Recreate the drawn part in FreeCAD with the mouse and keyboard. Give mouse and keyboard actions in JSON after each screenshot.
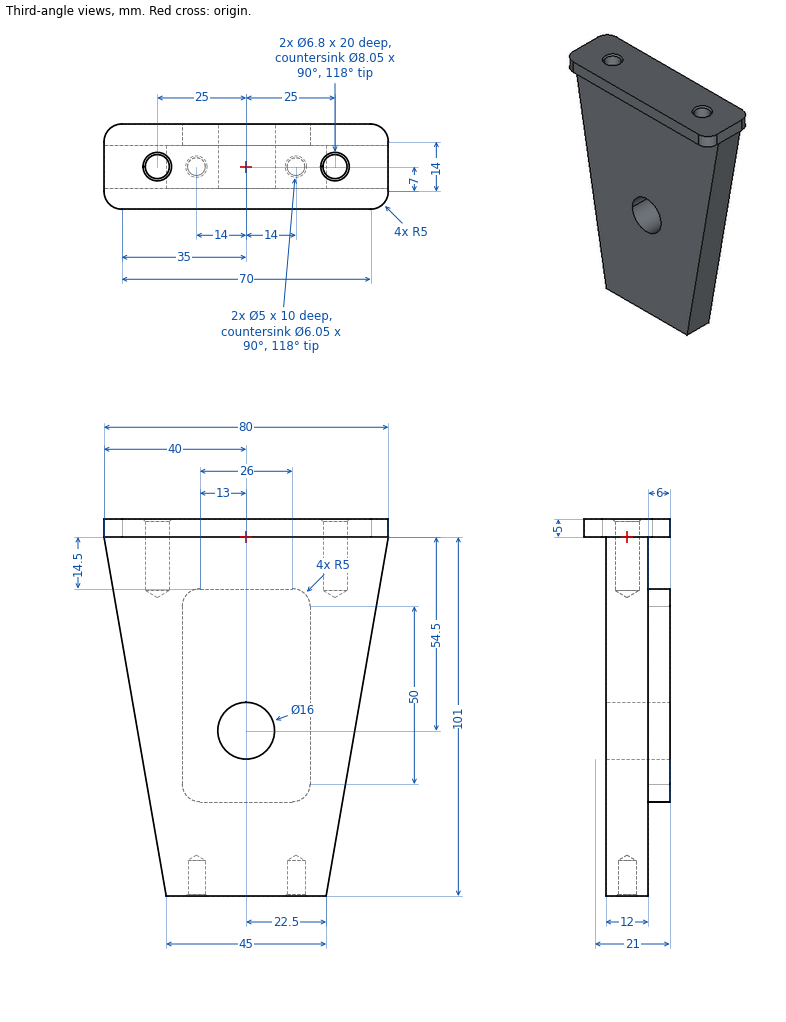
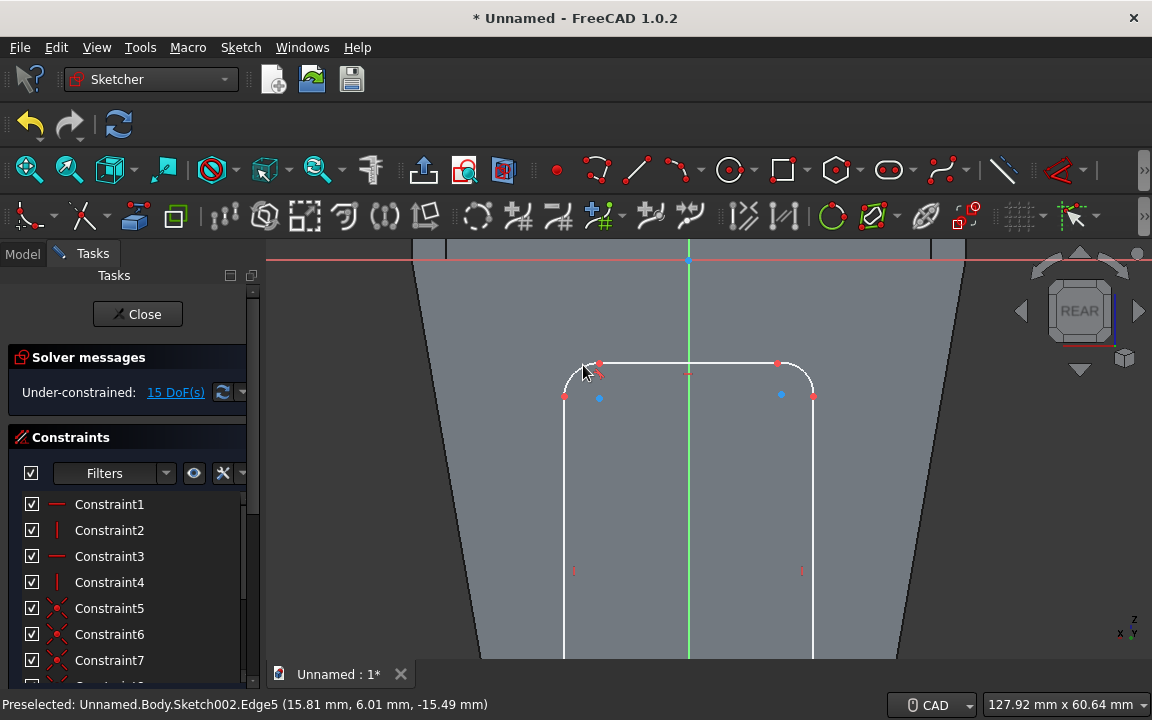
{"action": "left_click", "coordinate": [724, 363]}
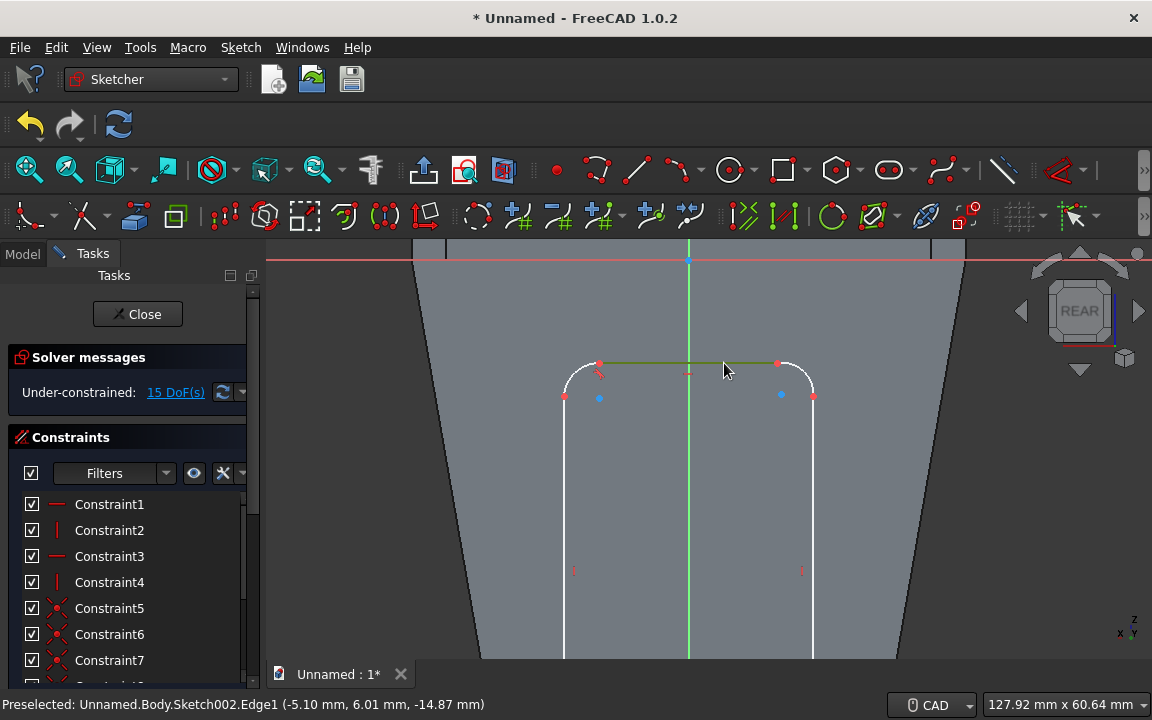
{"action": "left_click", "coordinate": [810, 380]}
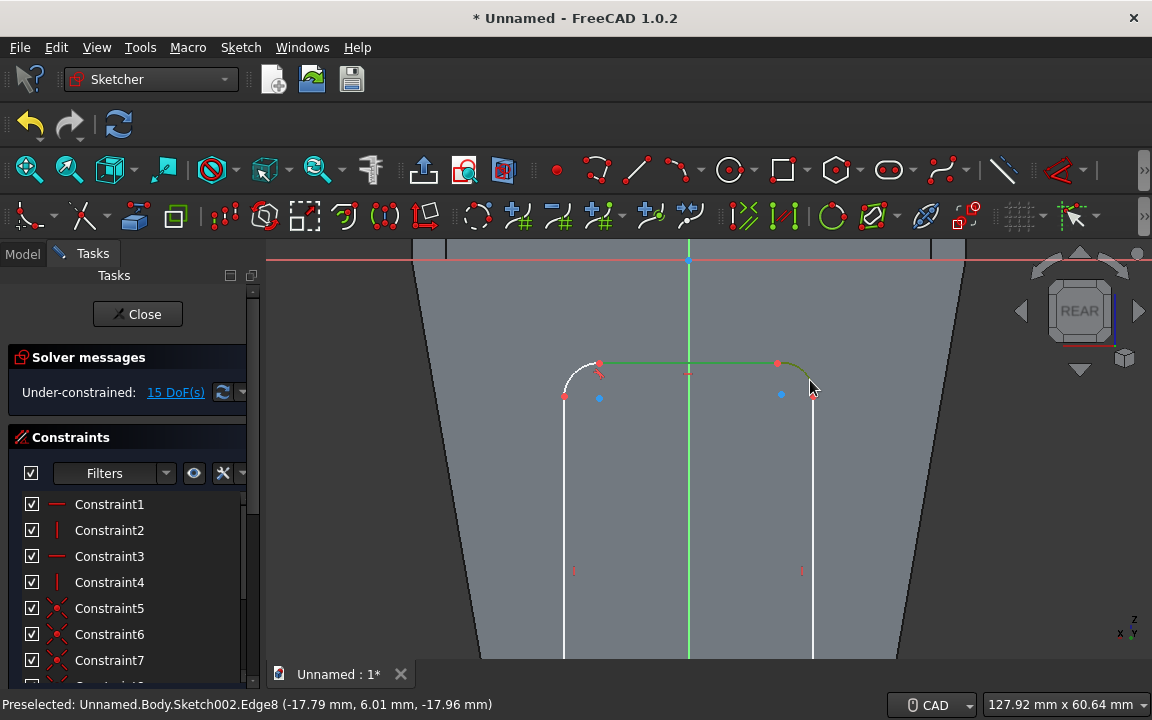
{"action": "key", "text": "t"}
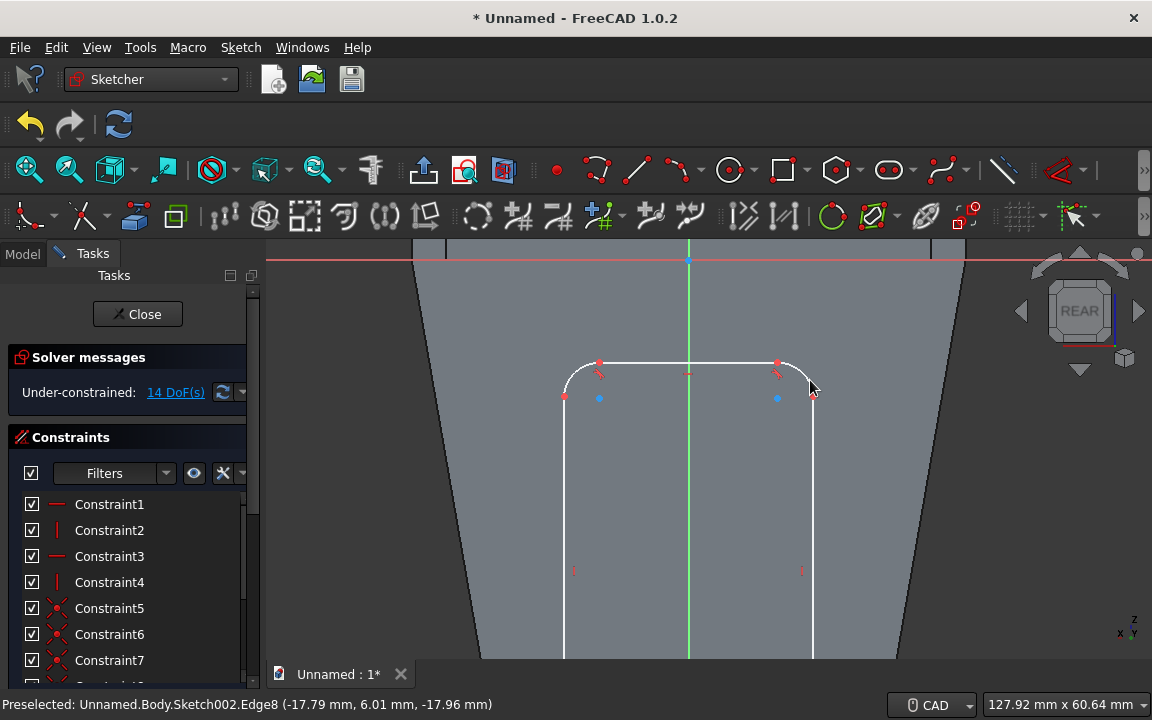
{"action": "left_click", "coordinate": [564, 501]}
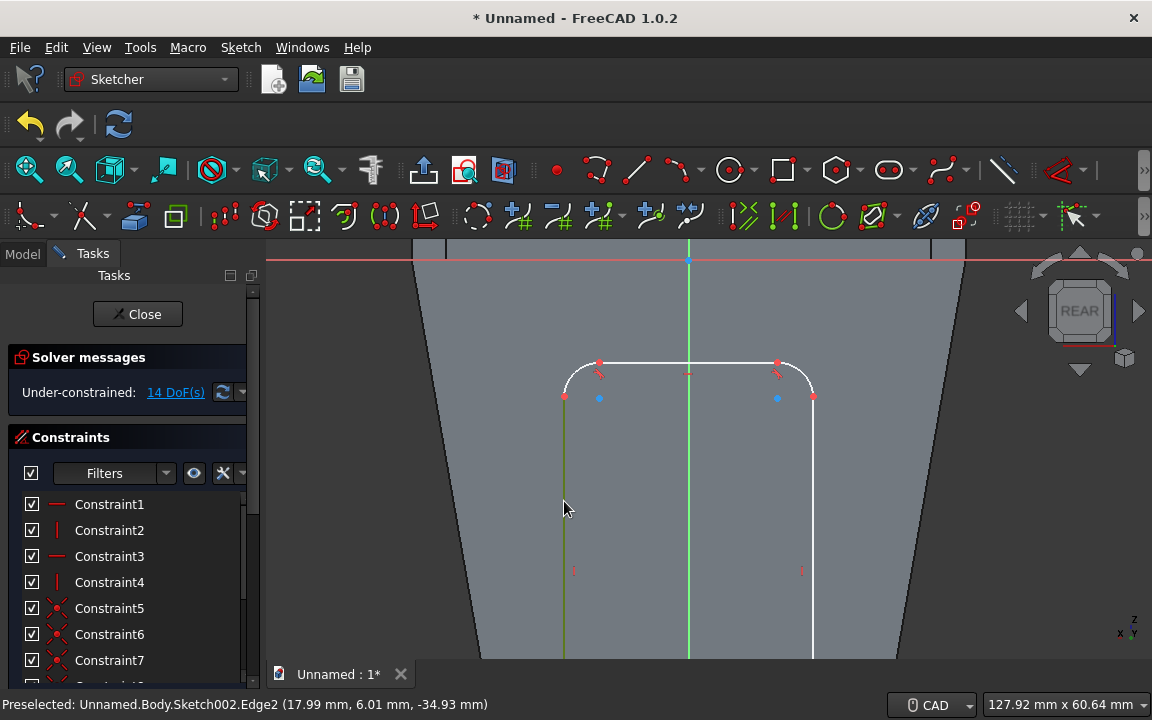
{"action": "left_click", "coordinate": [584, 366]}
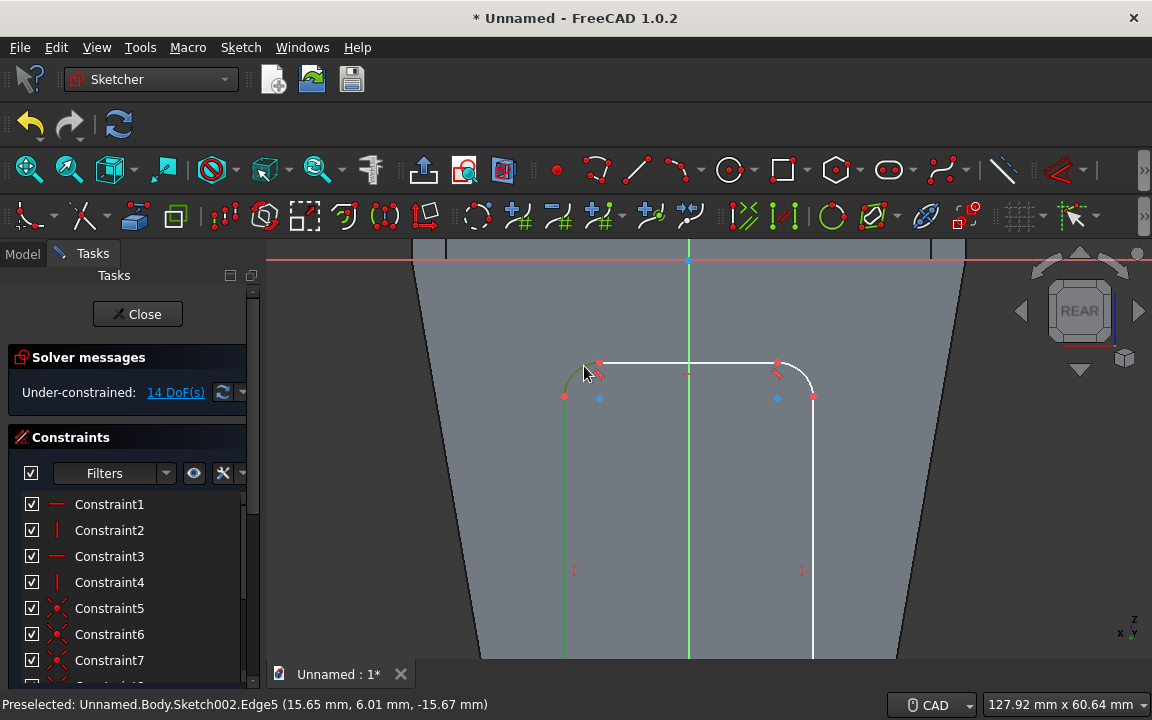
{"action": "key", "text": "t"}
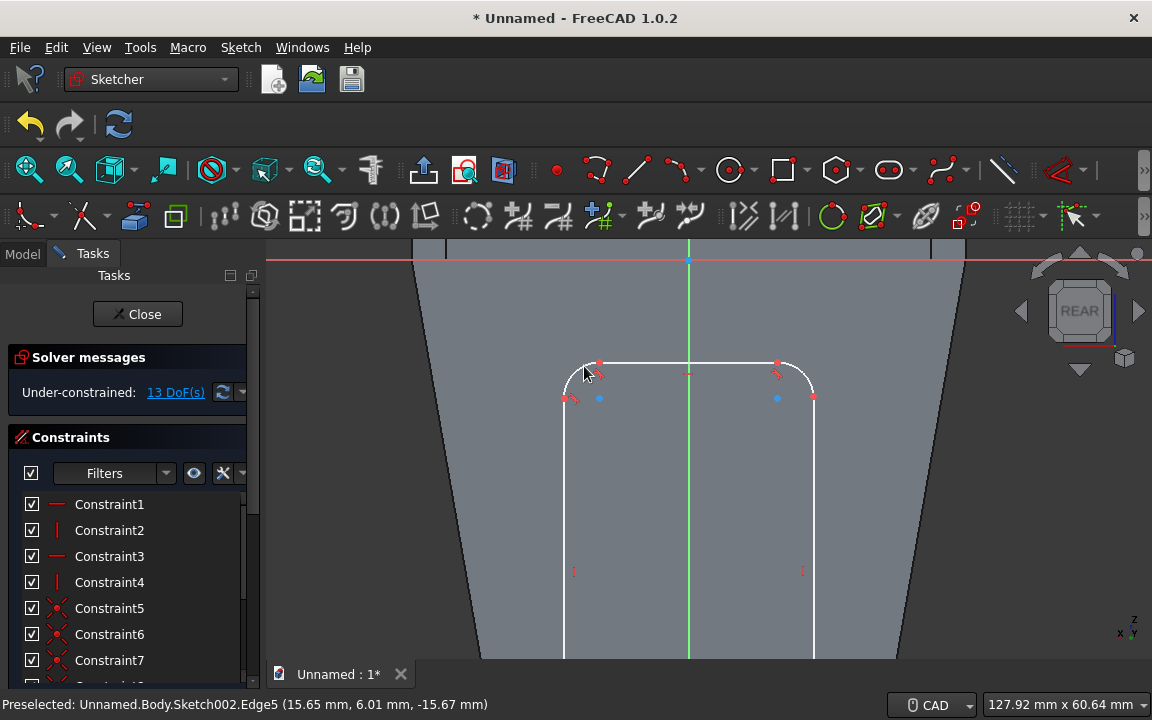
{"action": "left_click", "coordinate": [564, 502]}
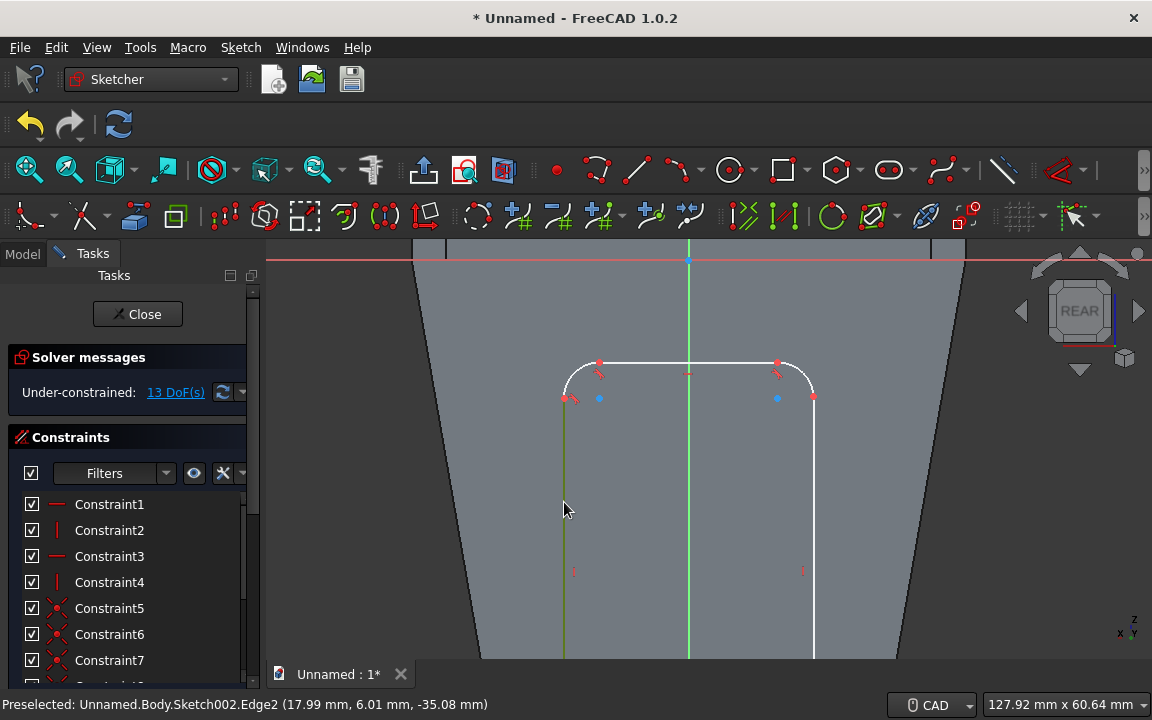
{"action": "scroll", "coordinate": [582, 365], "scroll_direction": "down", "scroll_amount": 3}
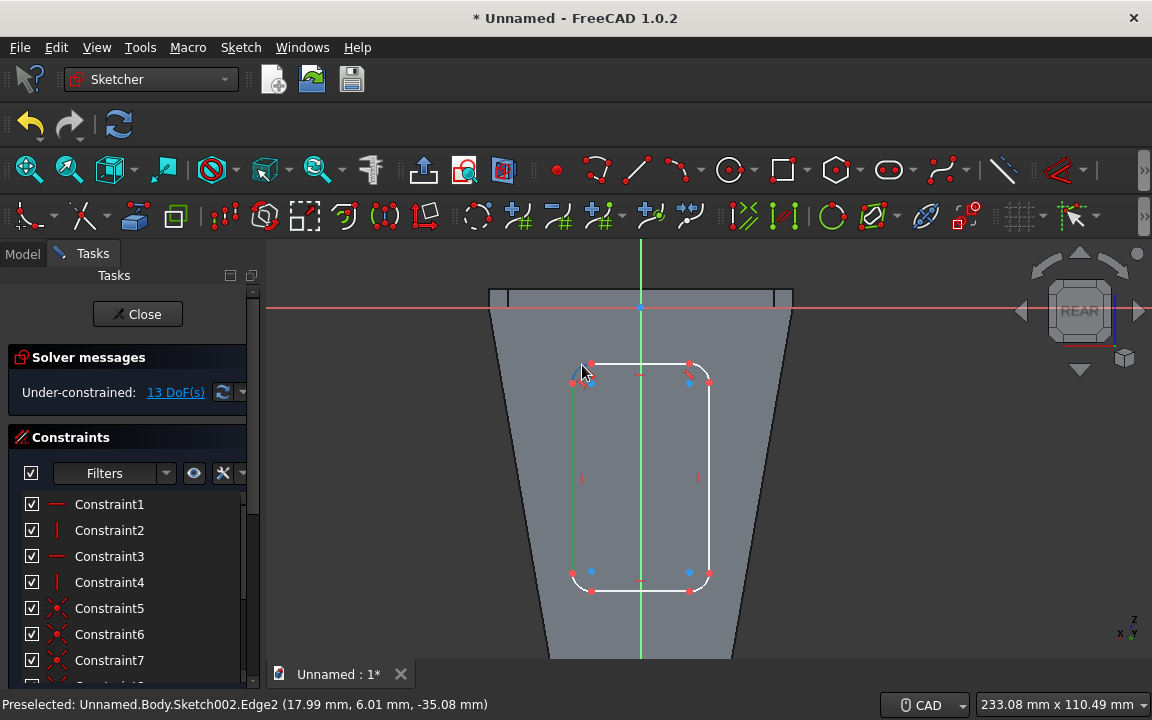
{"action": "scroll", "coordinate": [575, 581], "scroll_direction": "up", "scroll_amount": 3}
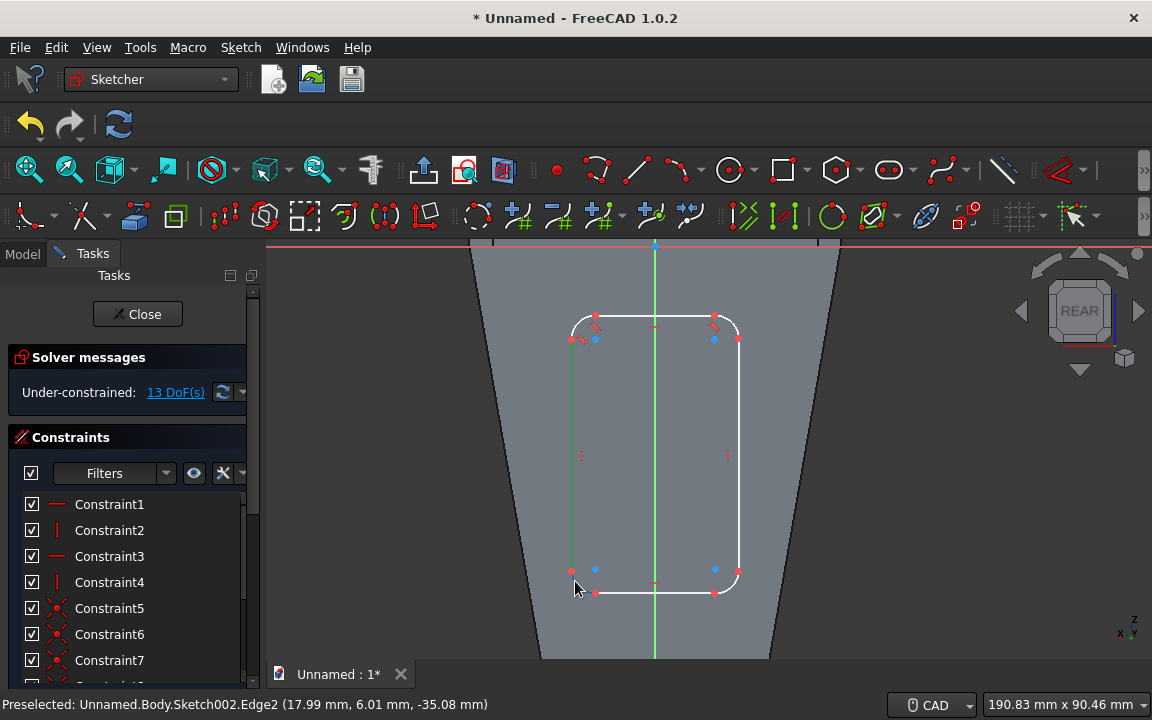
{"action": "left_click", "coordinate": [574, 581]}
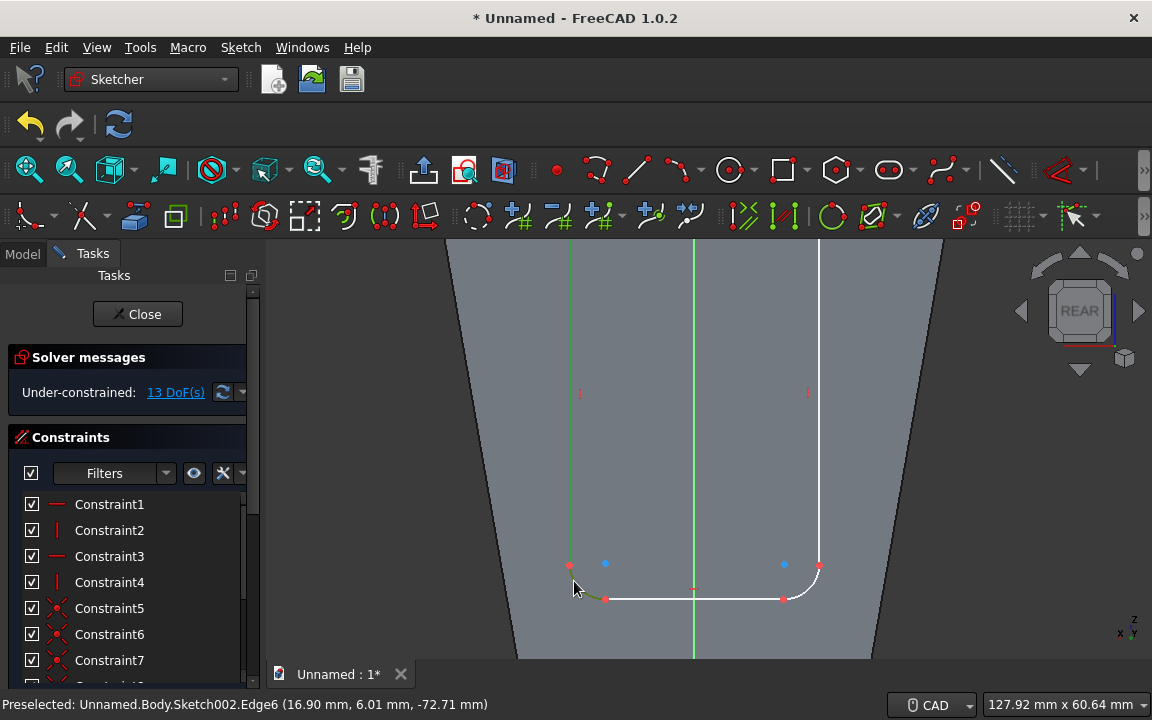
{"action": "key", "text": "t"}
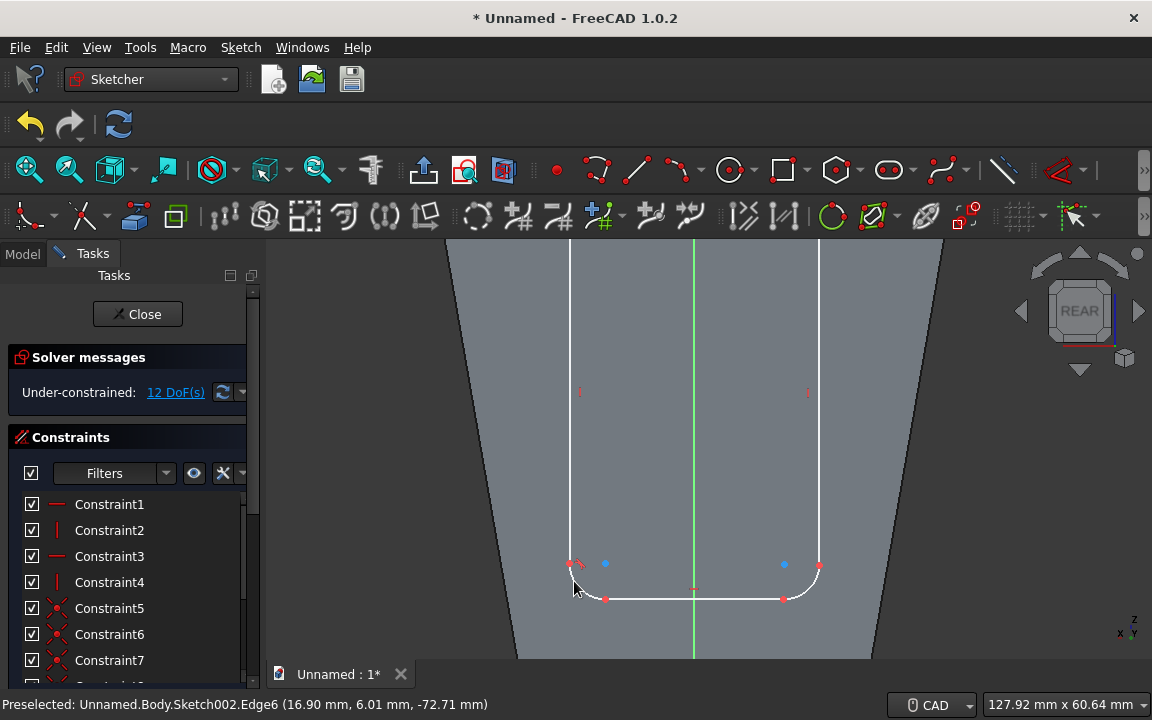
{"action": "left_click", "coordinate": [659, 599]}